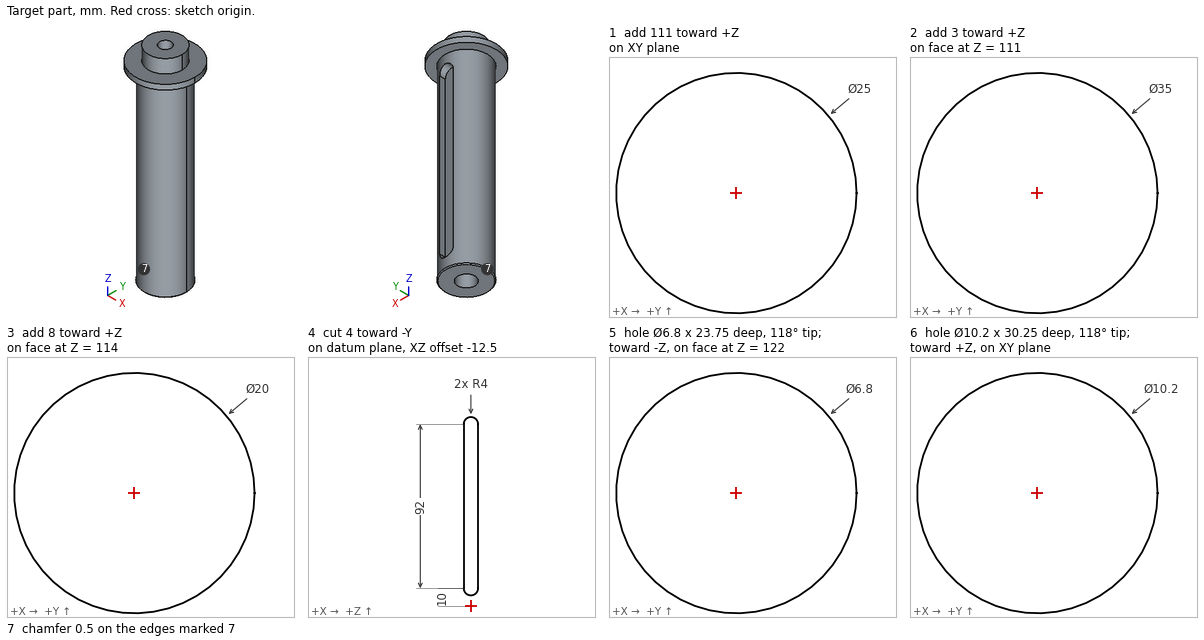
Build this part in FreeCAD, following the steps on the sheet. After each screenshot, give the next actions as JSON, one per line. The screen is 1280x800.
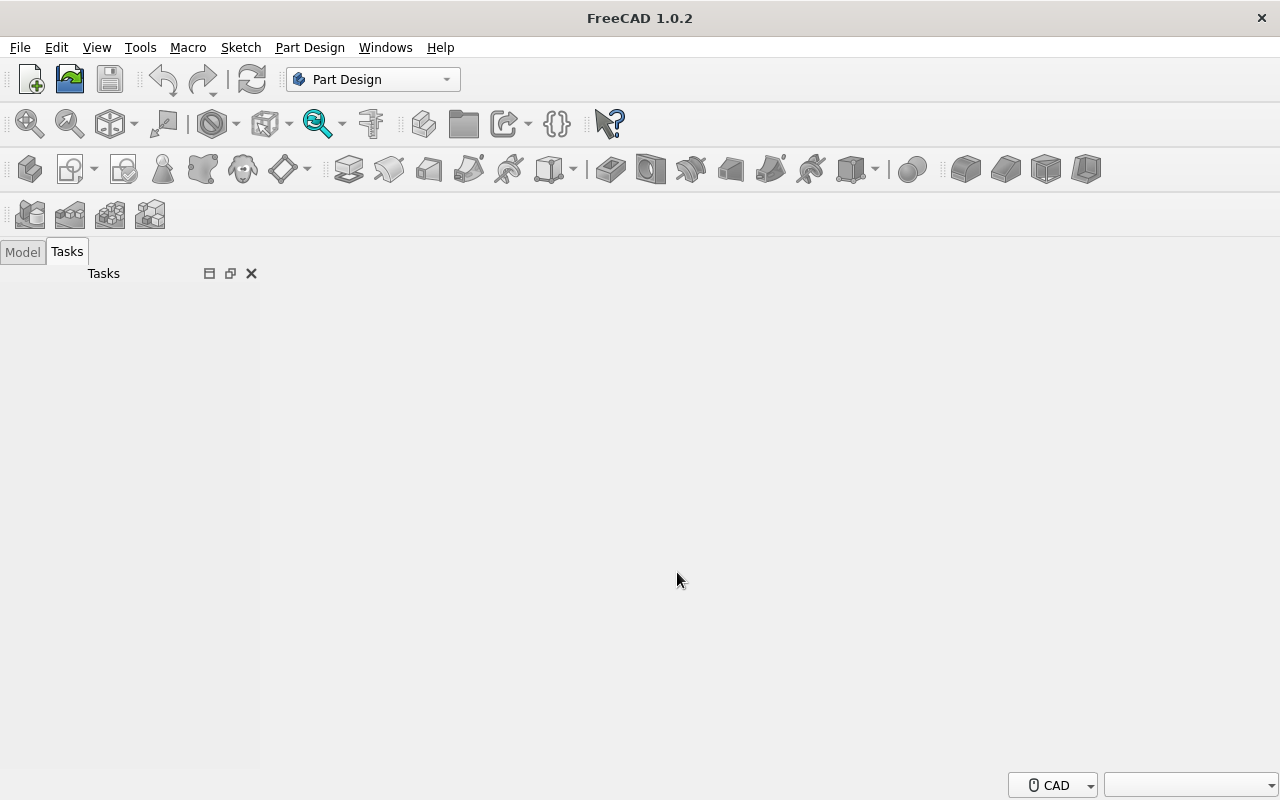
{"action": "left_click", "coordinate": [30, 80]}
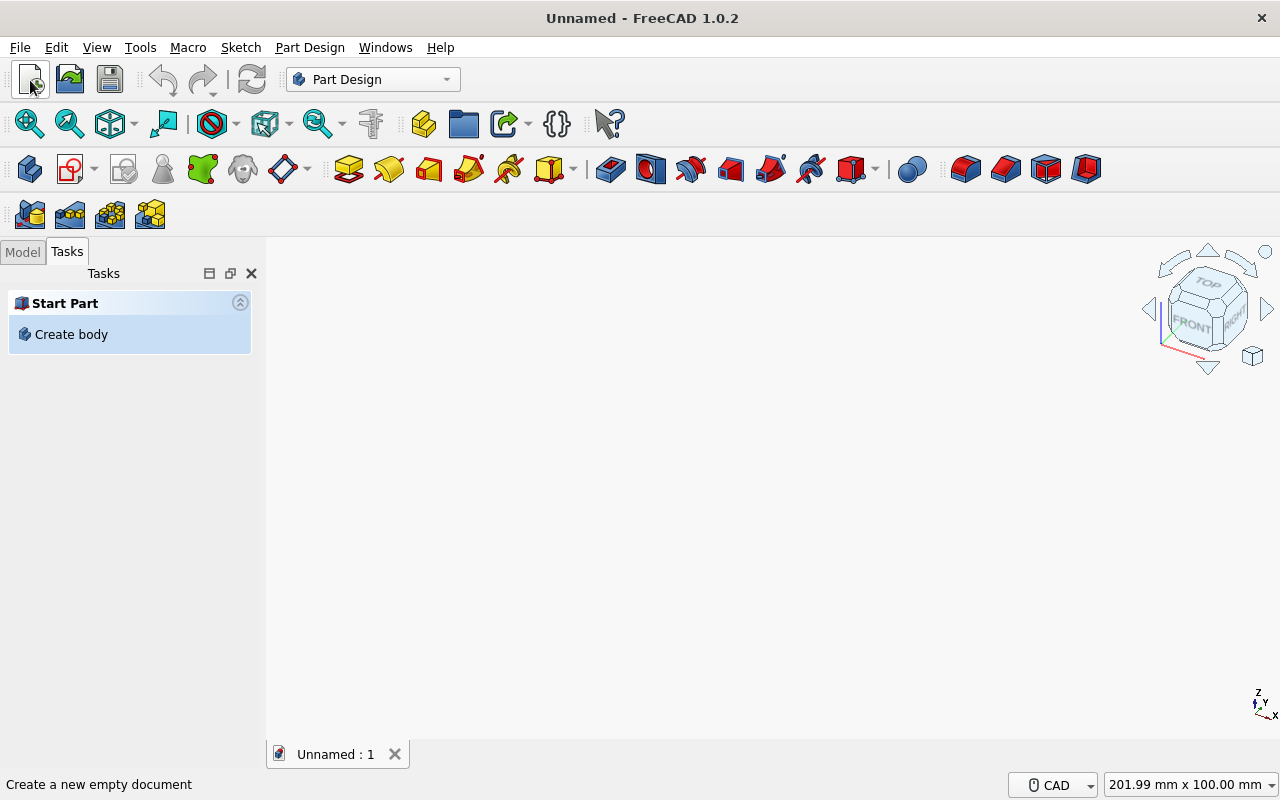
{"action": "left_click", "coordinate": [70, 170]}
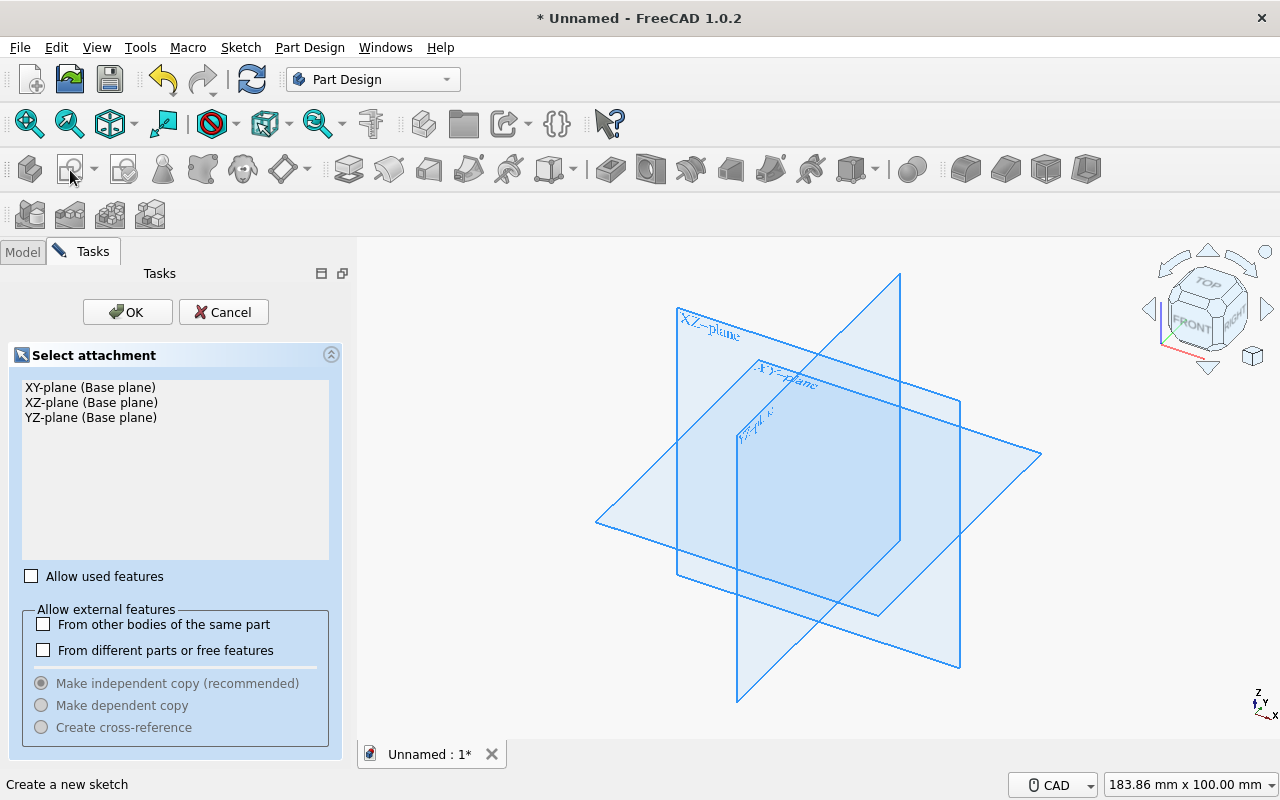
{"action": "left_click", "coordinate": [82, 388]}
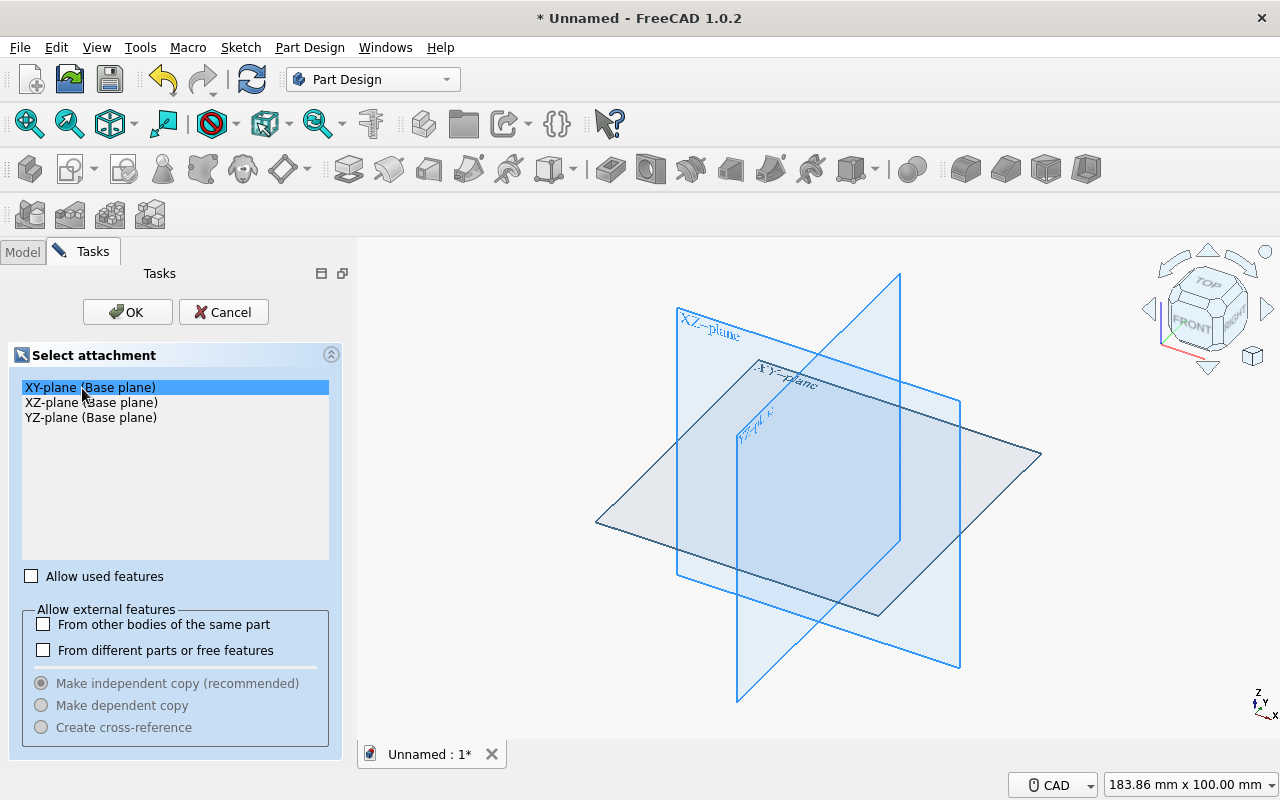
{"action": "left_click", "coordinate": [128, 312]}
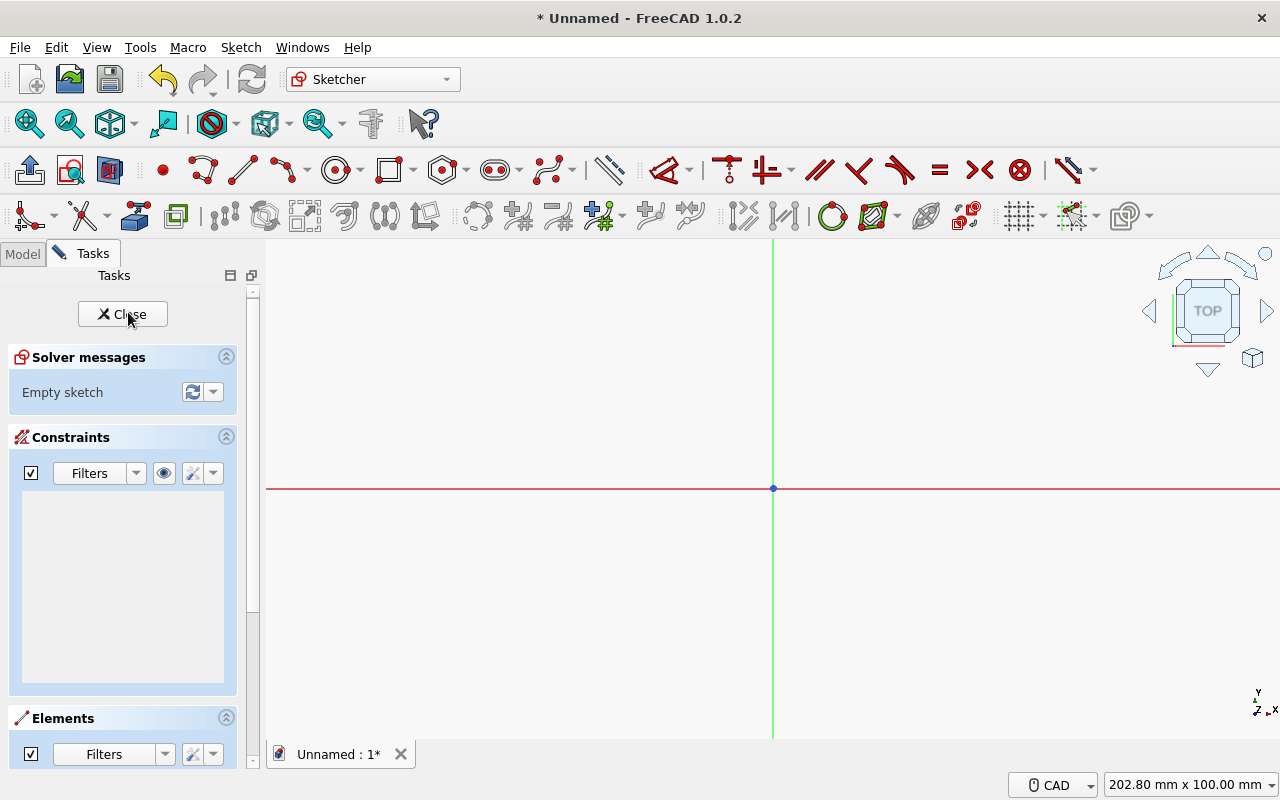
{"action": "scroll", "coordinate": [813, 489], "scroll_direction": "up", "scroll_amount": 5}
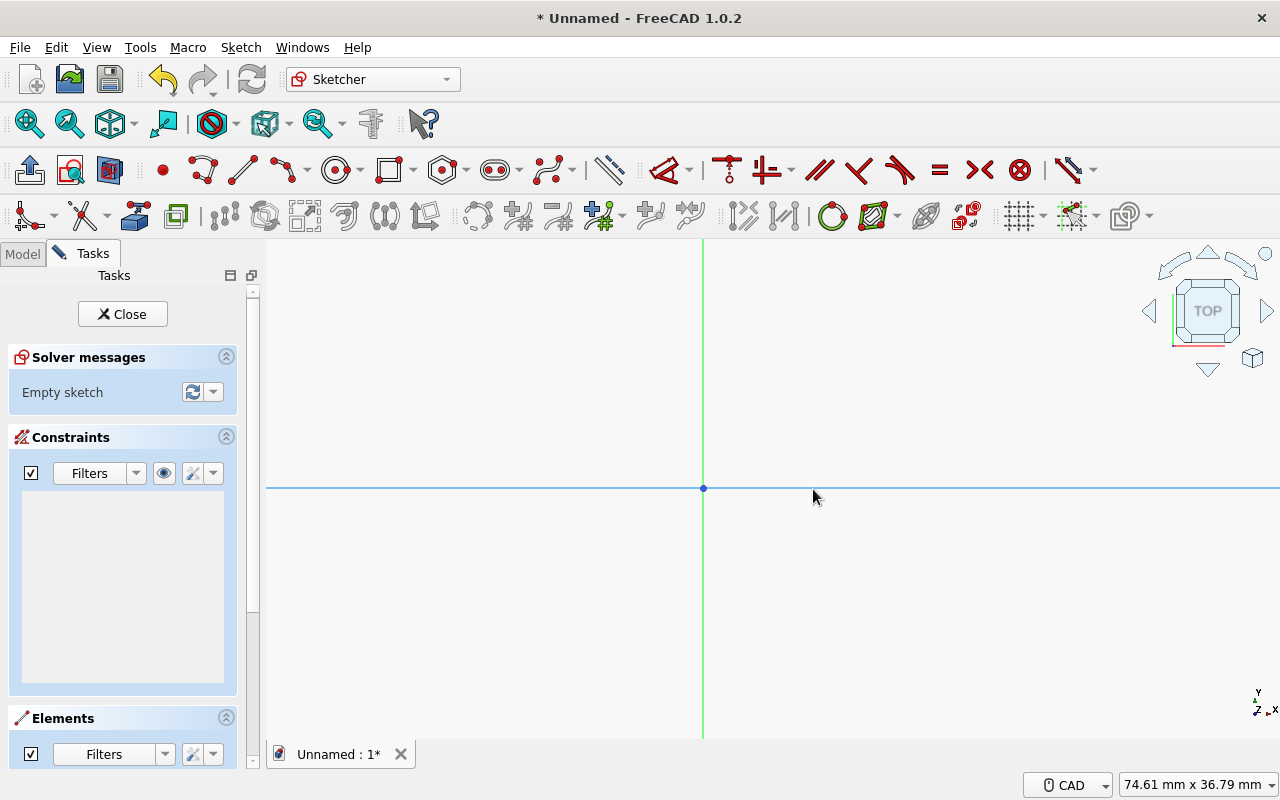
{"action": "left_click", "coordinate": [336, 170]}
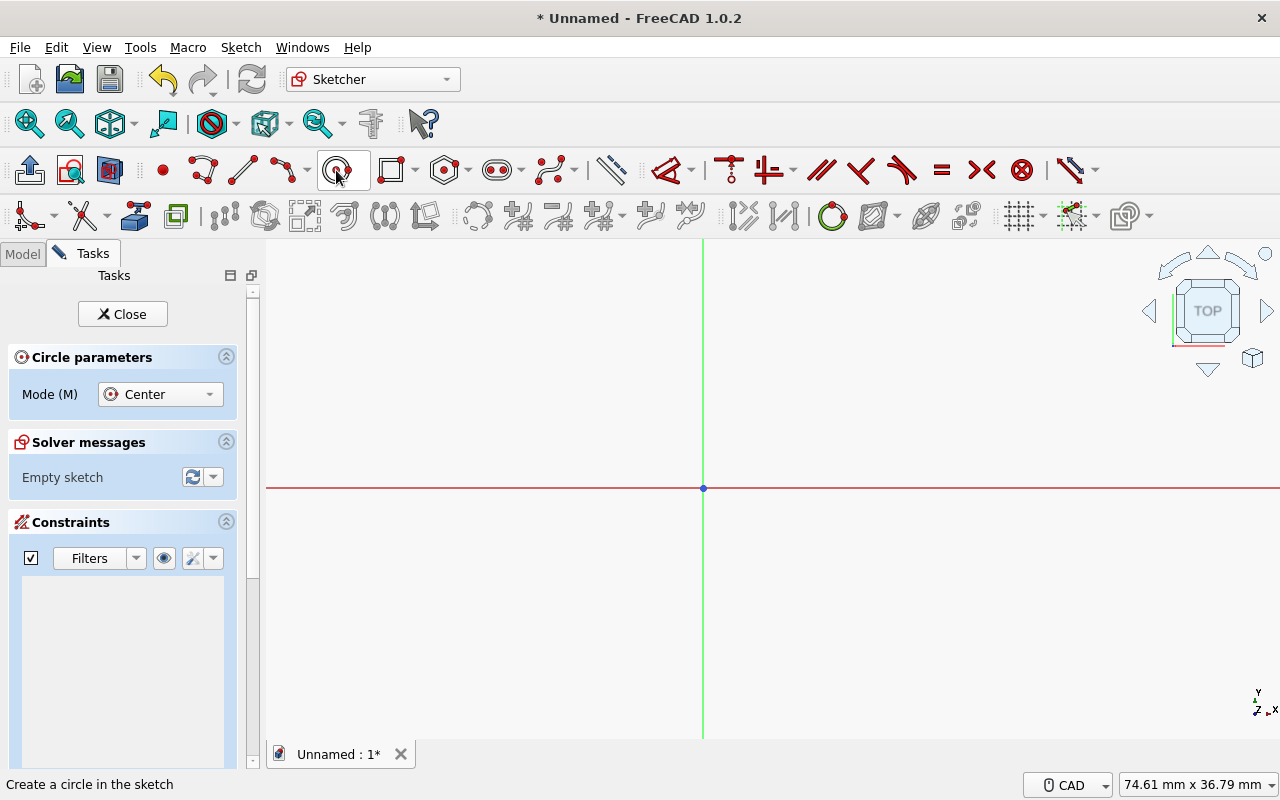
{"action": "left_click", "coordinate": [703, 488]}
{"action": "mouse_move", "coordinate": [823, 368]}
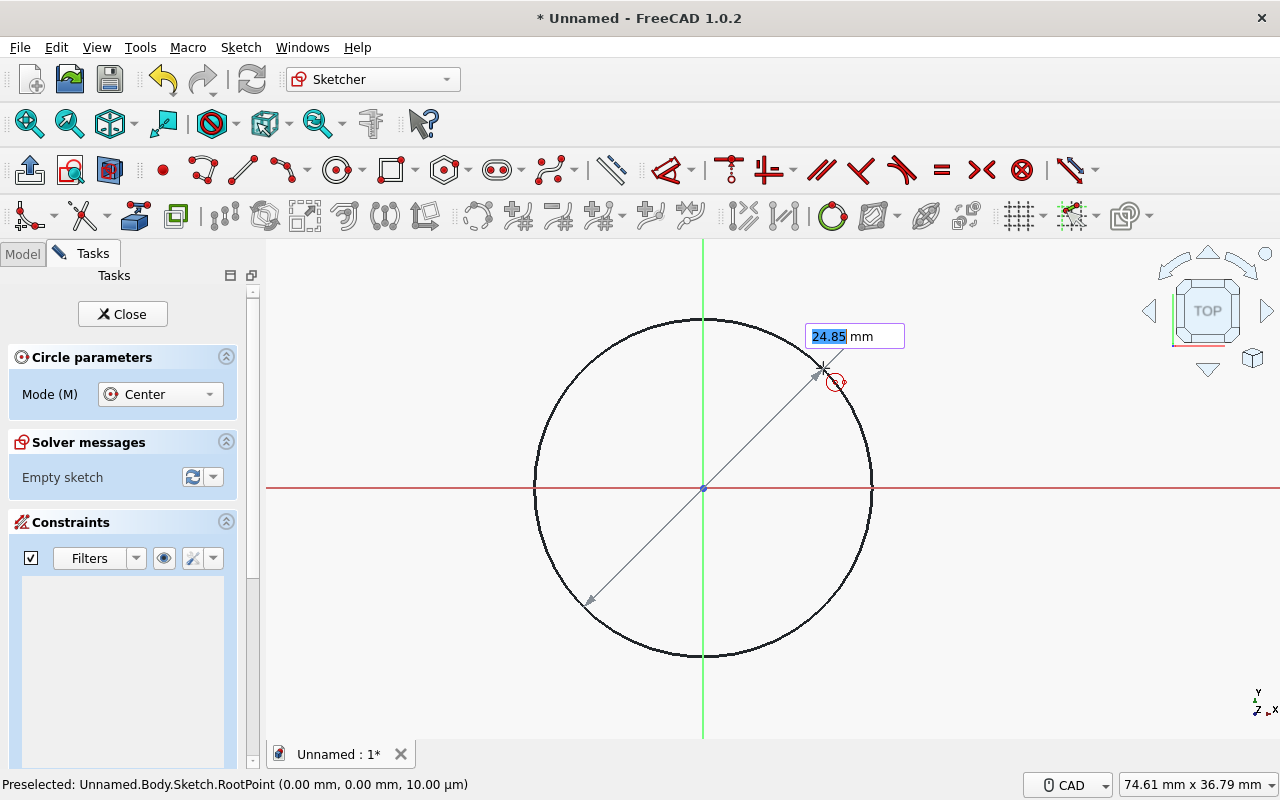
{"action": "type", "text": "25"}
{"action": "key", "text": "Return"}
{"action": "key", "text": "Escape"}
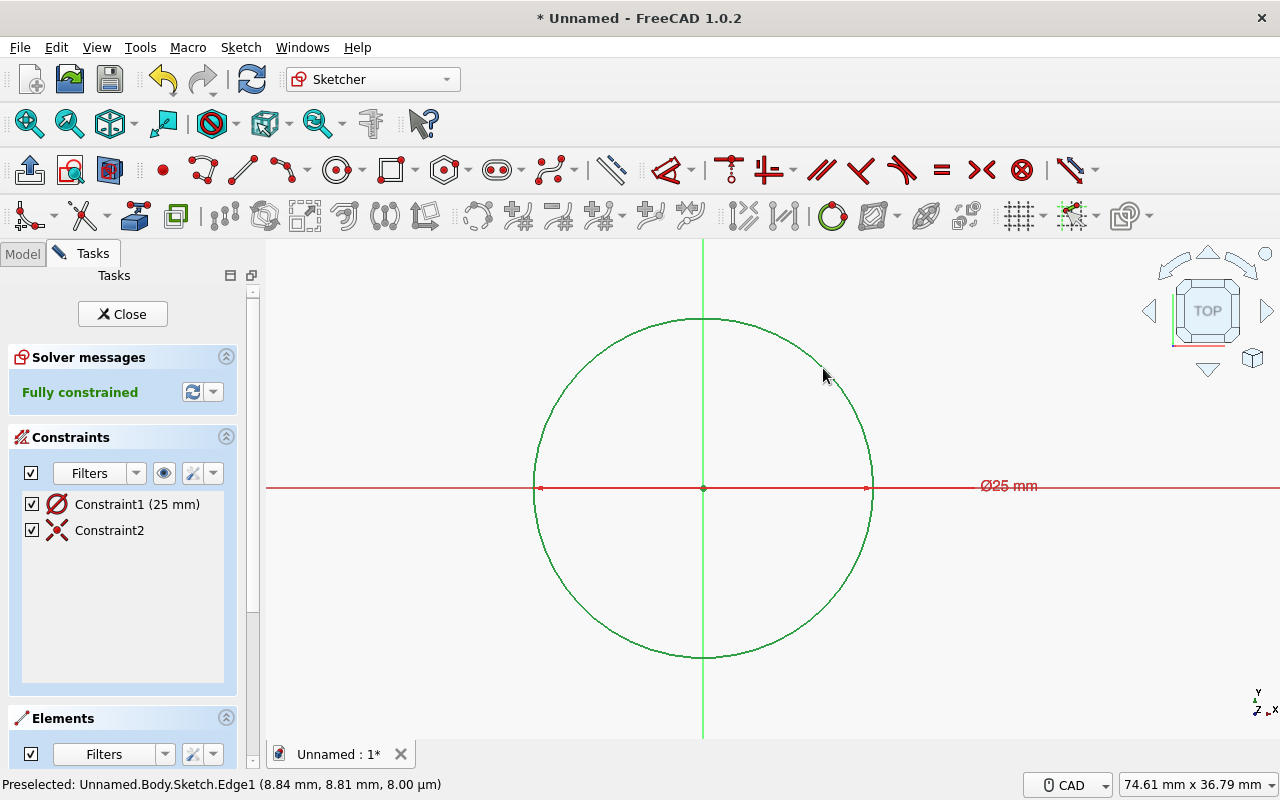
{"action": "left_click", "coordinate": [123, 314]}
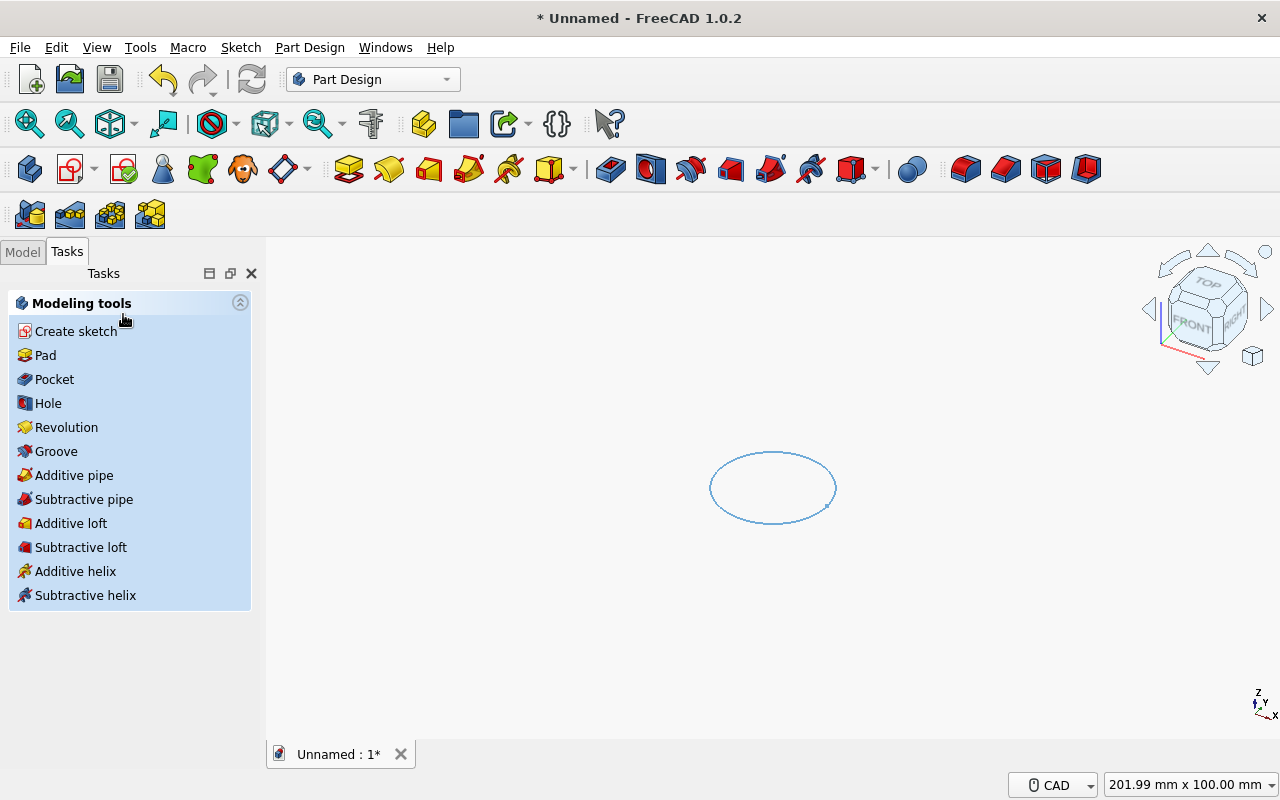
{"action": "left_click", "coordinate": [350, 170]}